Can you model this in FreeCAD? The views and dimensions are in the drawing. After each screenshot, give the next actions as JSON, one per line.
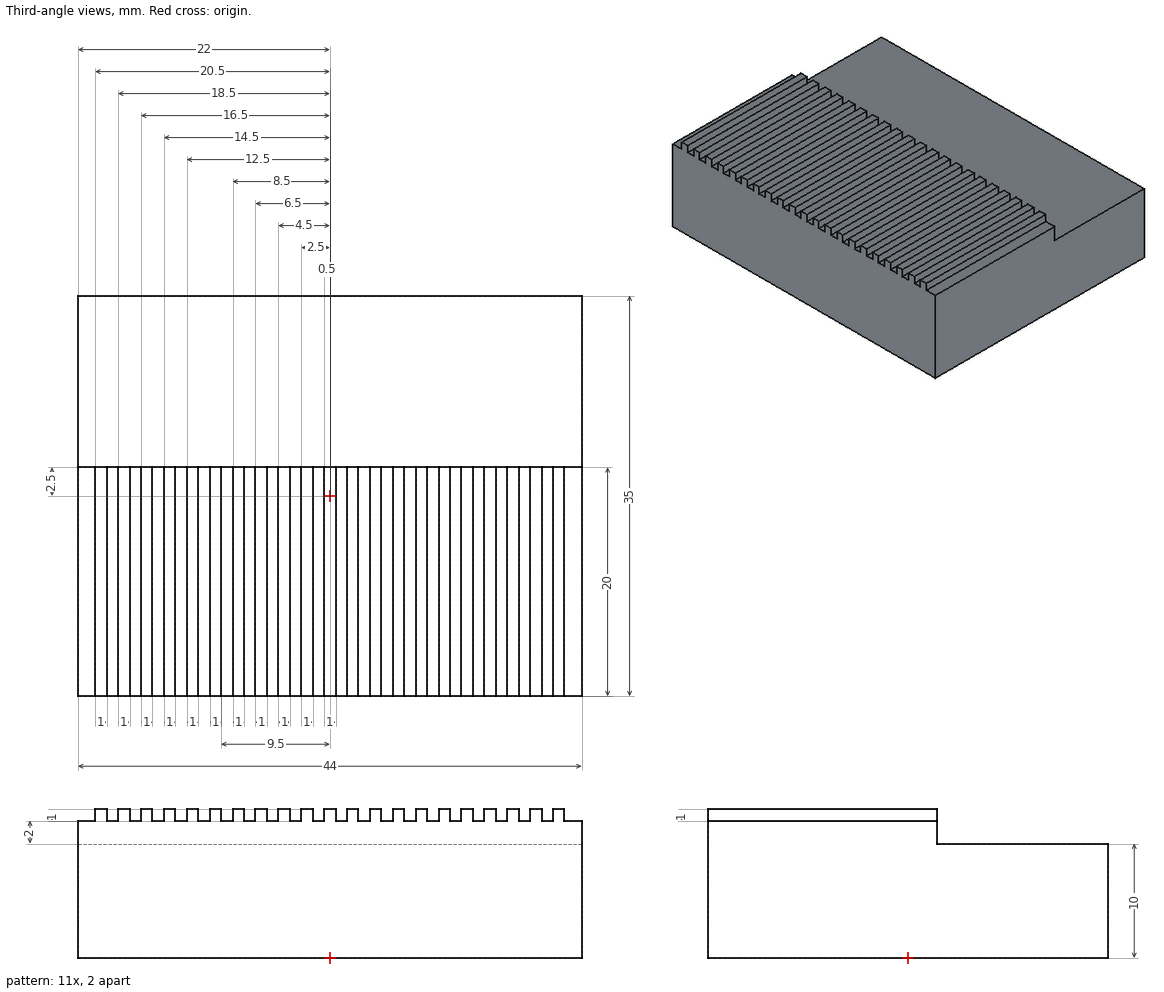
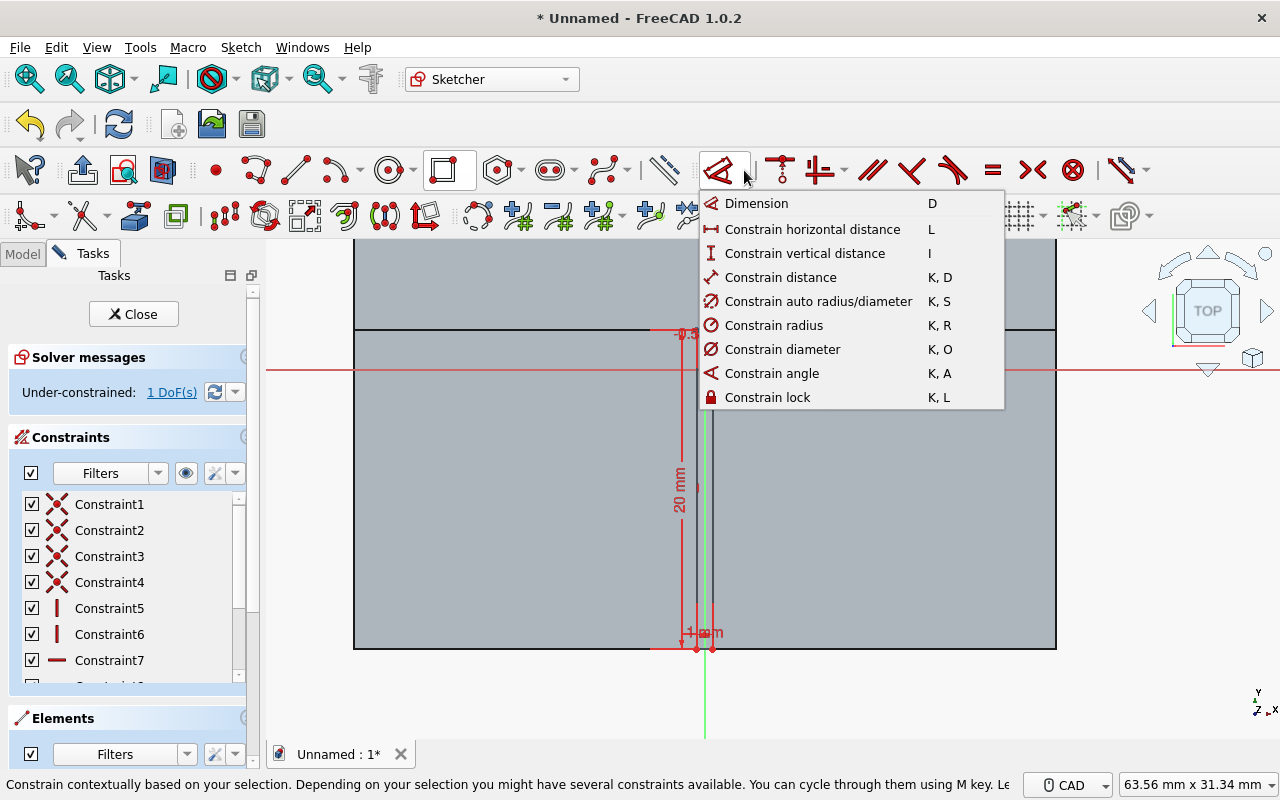
{"action": "left_click", "coordinate": [852, 253]}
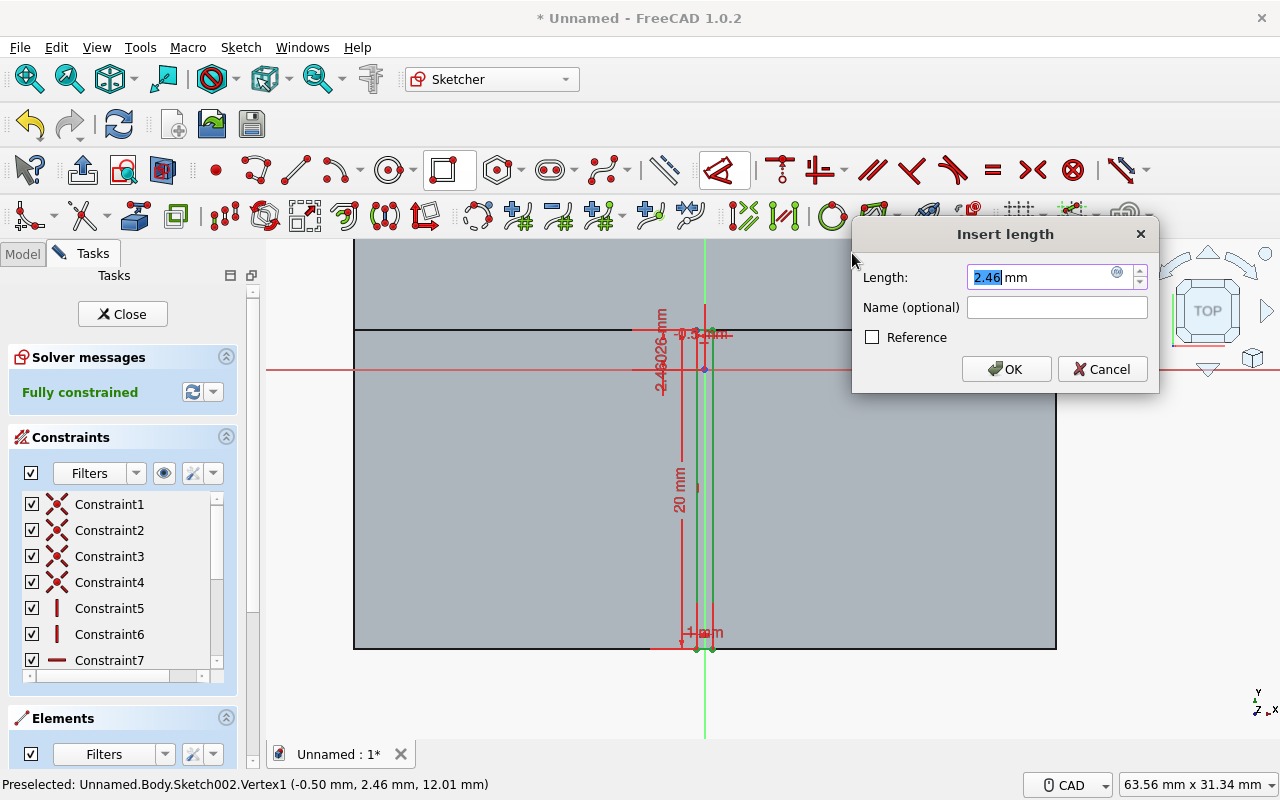
{"action": "type", "text": "2.5"}
{"action": "key", "text": "Return"}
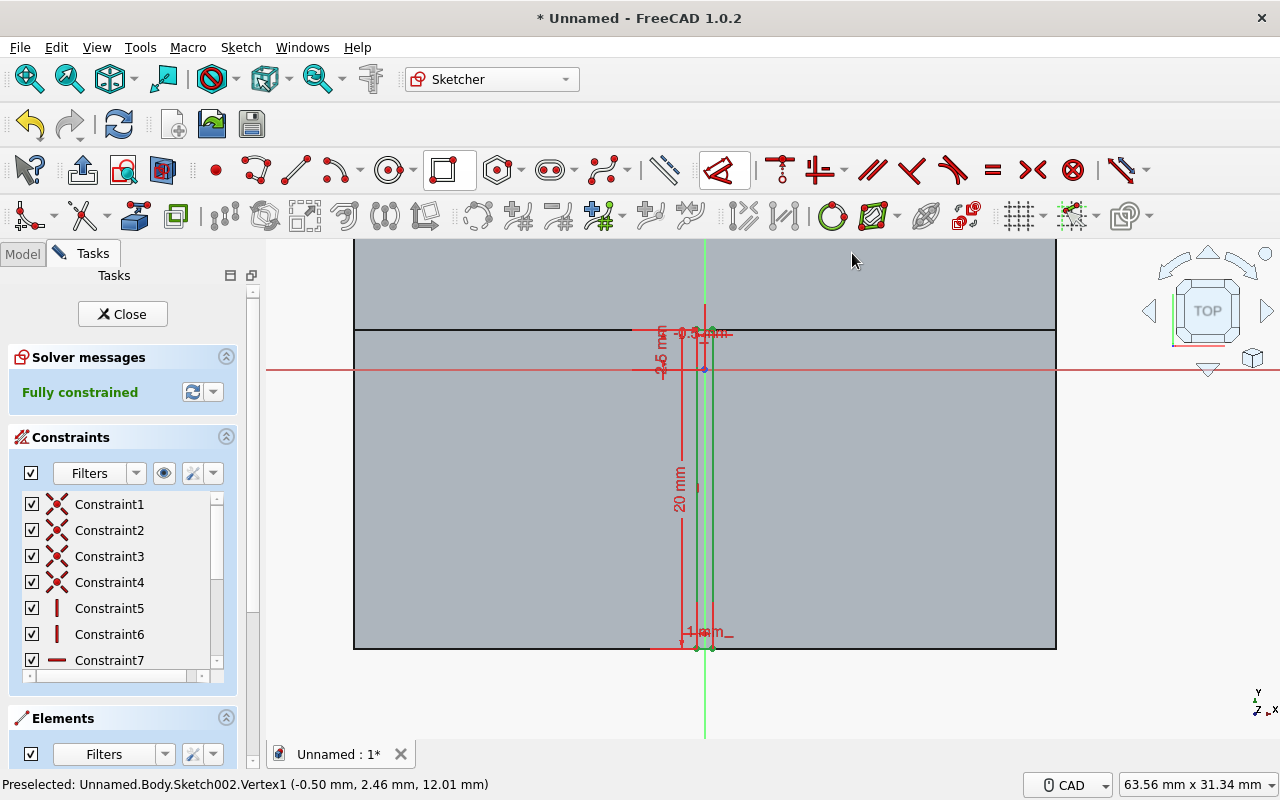
{"action": "left_click", "coordinate": [123, 314]}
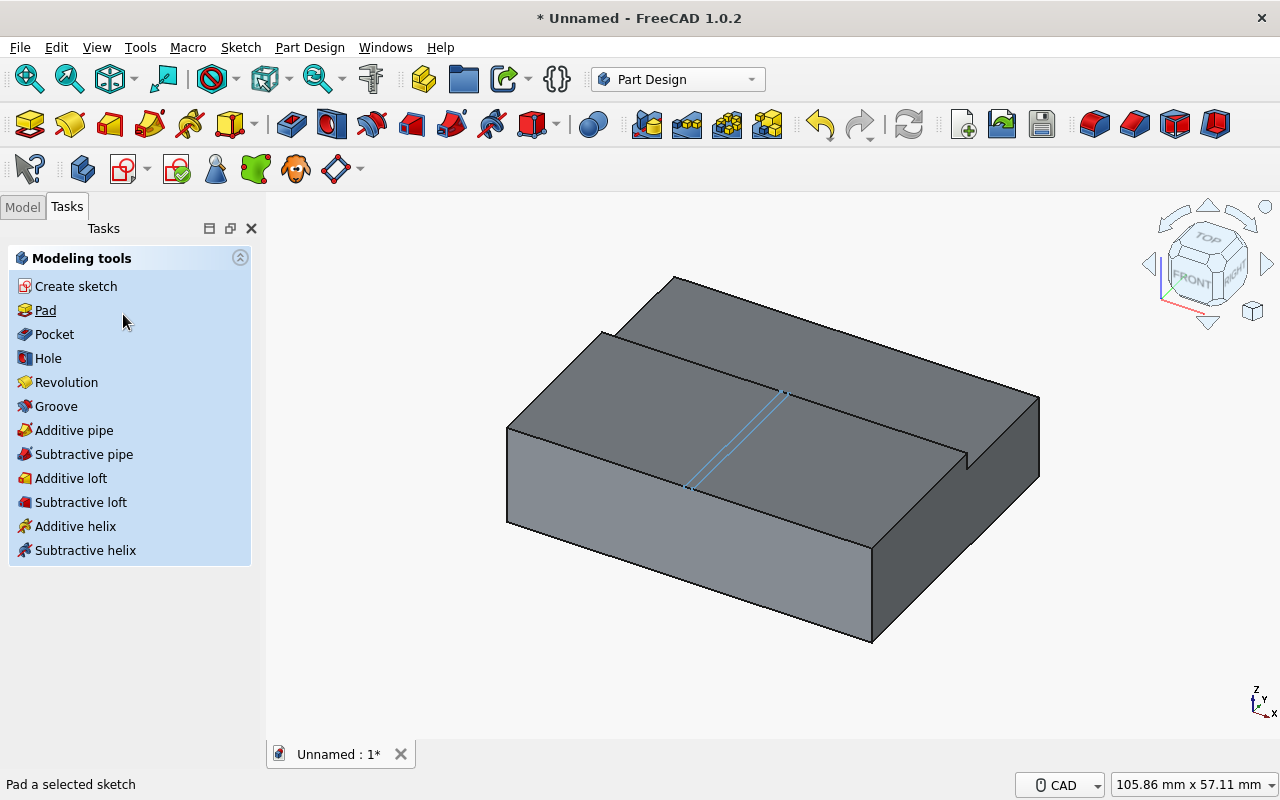
{"action": "left_click", "coordinate": [30, 124]}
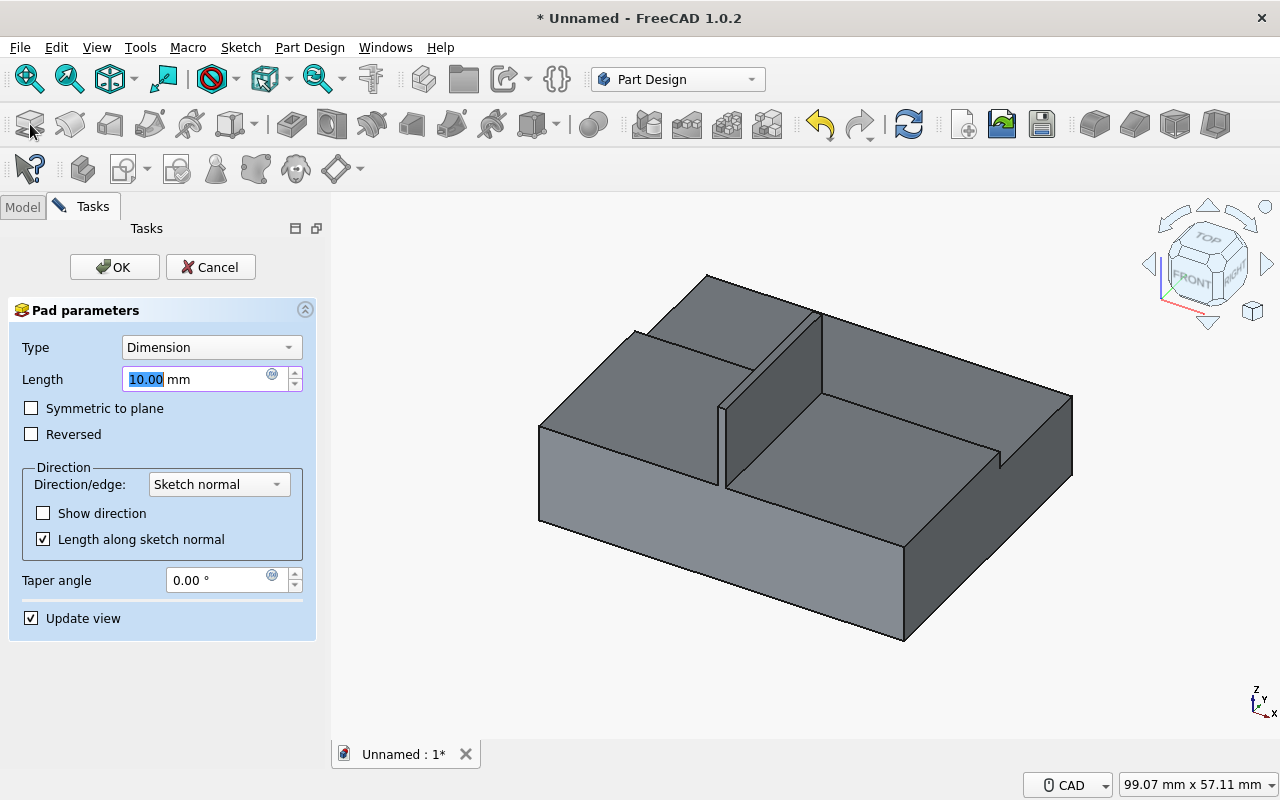
{"action": "type", "text": "1"}
{"action": "key", "text": "Tab"}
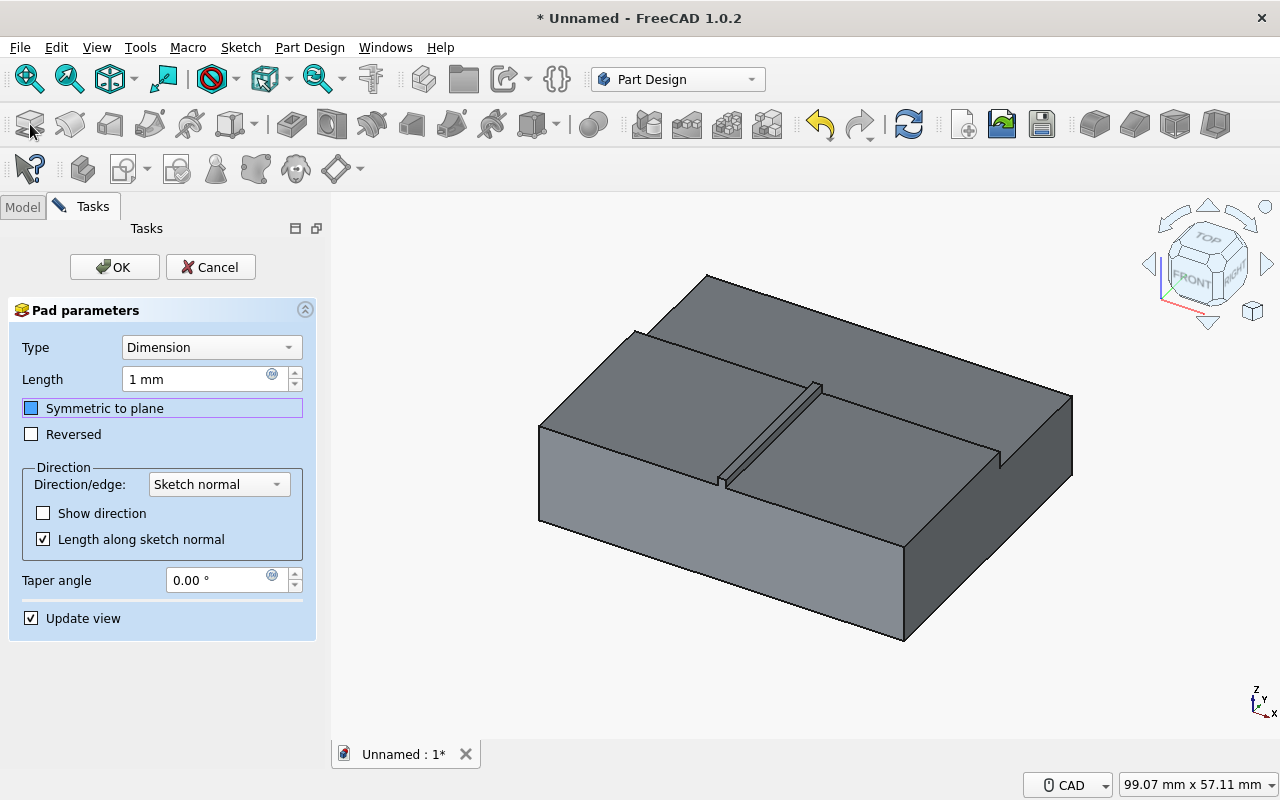
{"action": "left_click", "coordinate": [115, 267]}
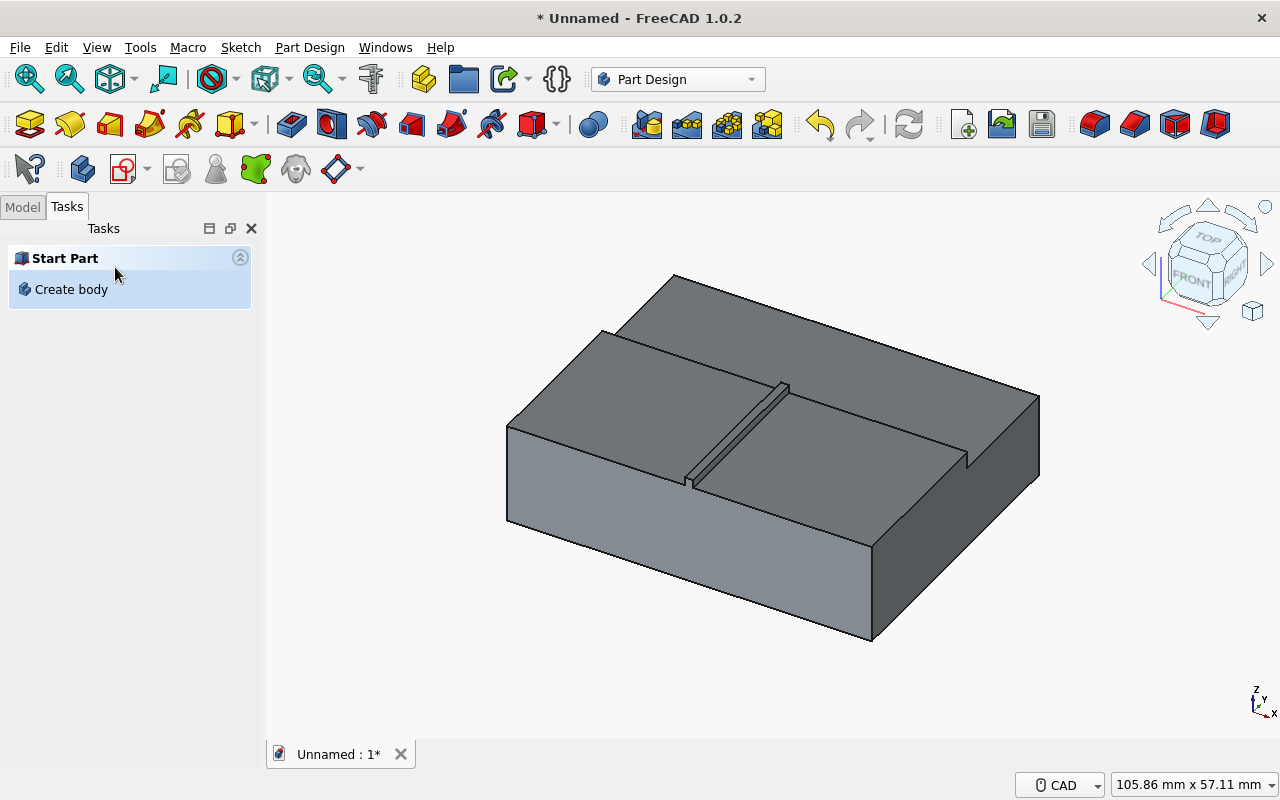
{"action": "left_click", "coordinate": [23, 206]}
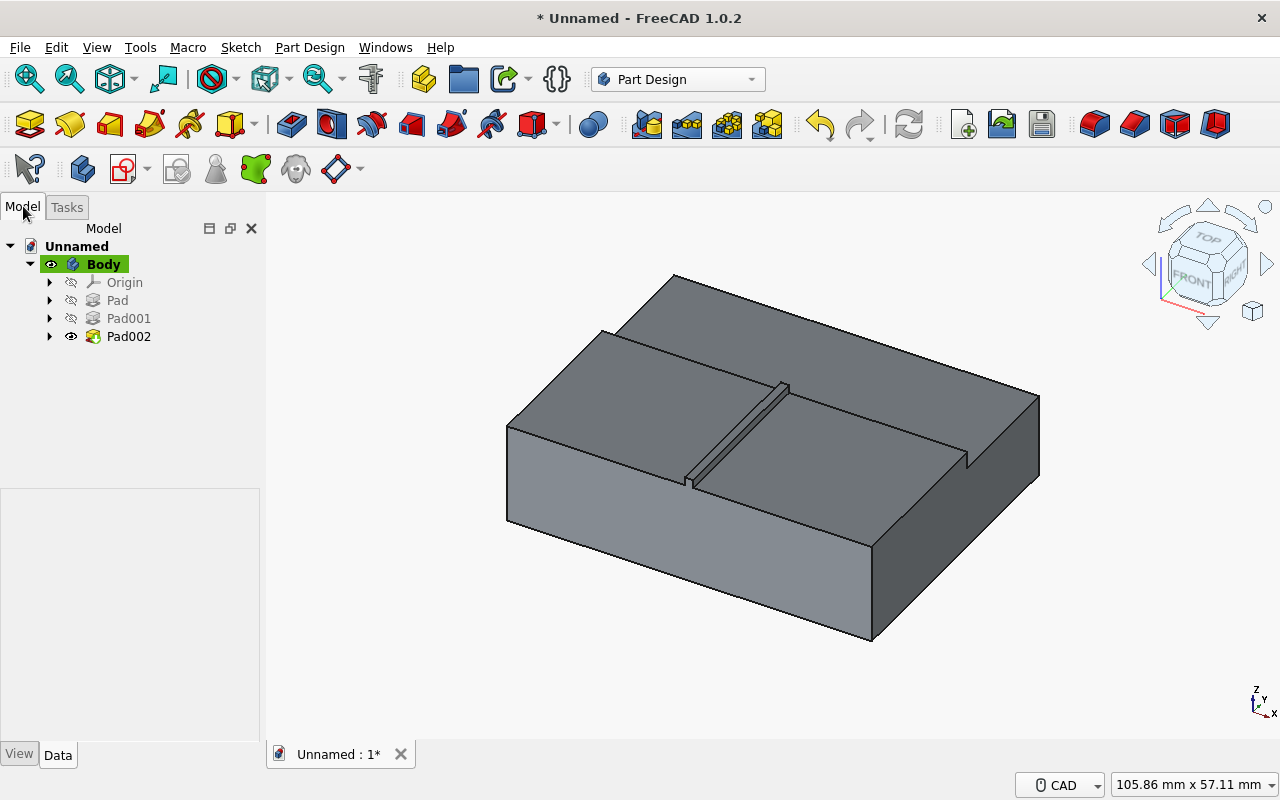
{"action": "left_click", "coordinate": [116, 336]}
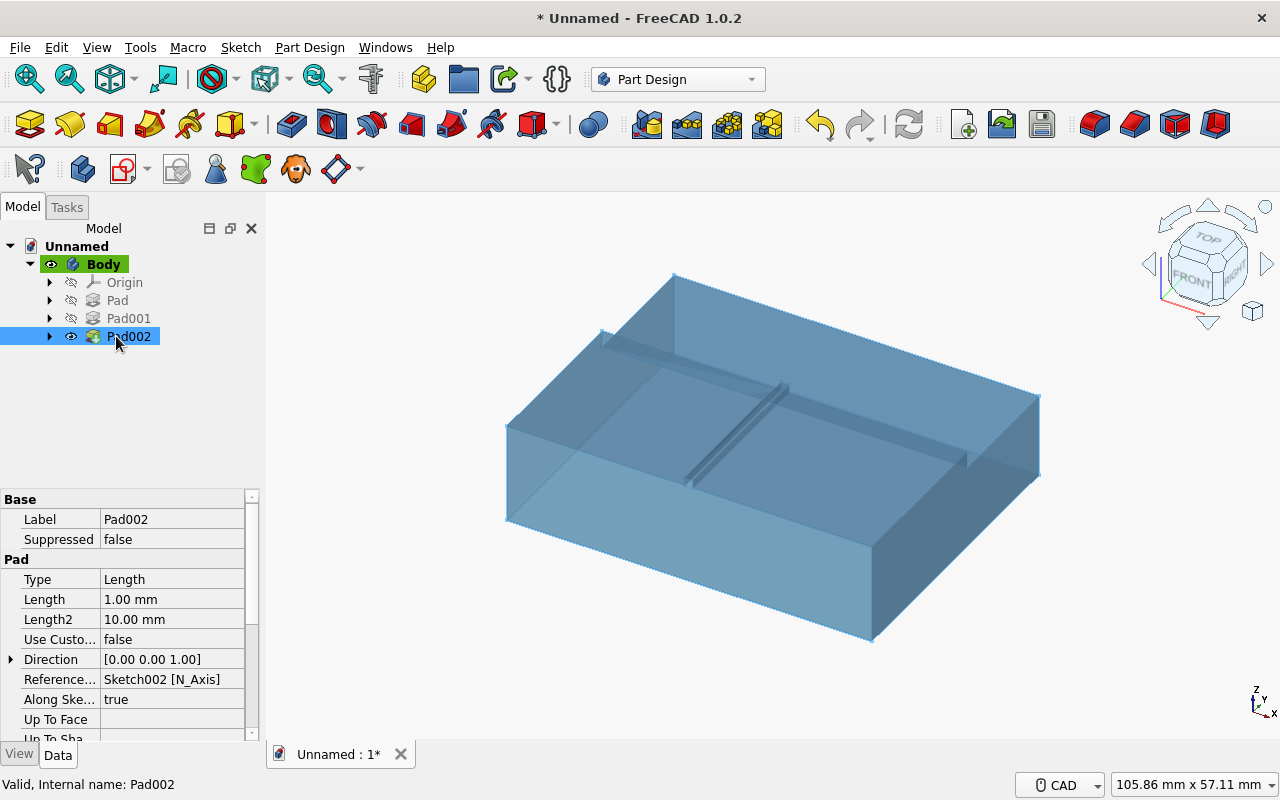
{"action": "left_click", "coordinate": [688, 124]}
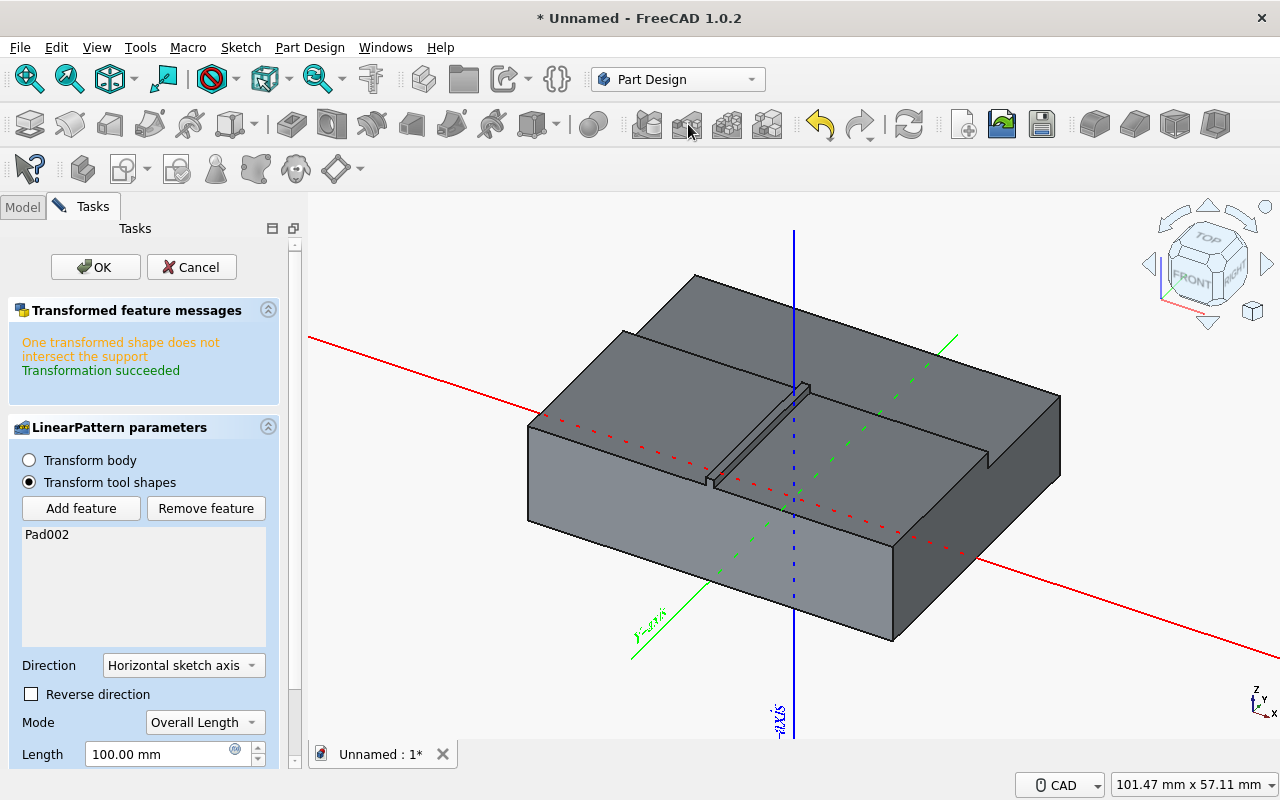
{"action": "left_click", "coordinate": [184, 666]}